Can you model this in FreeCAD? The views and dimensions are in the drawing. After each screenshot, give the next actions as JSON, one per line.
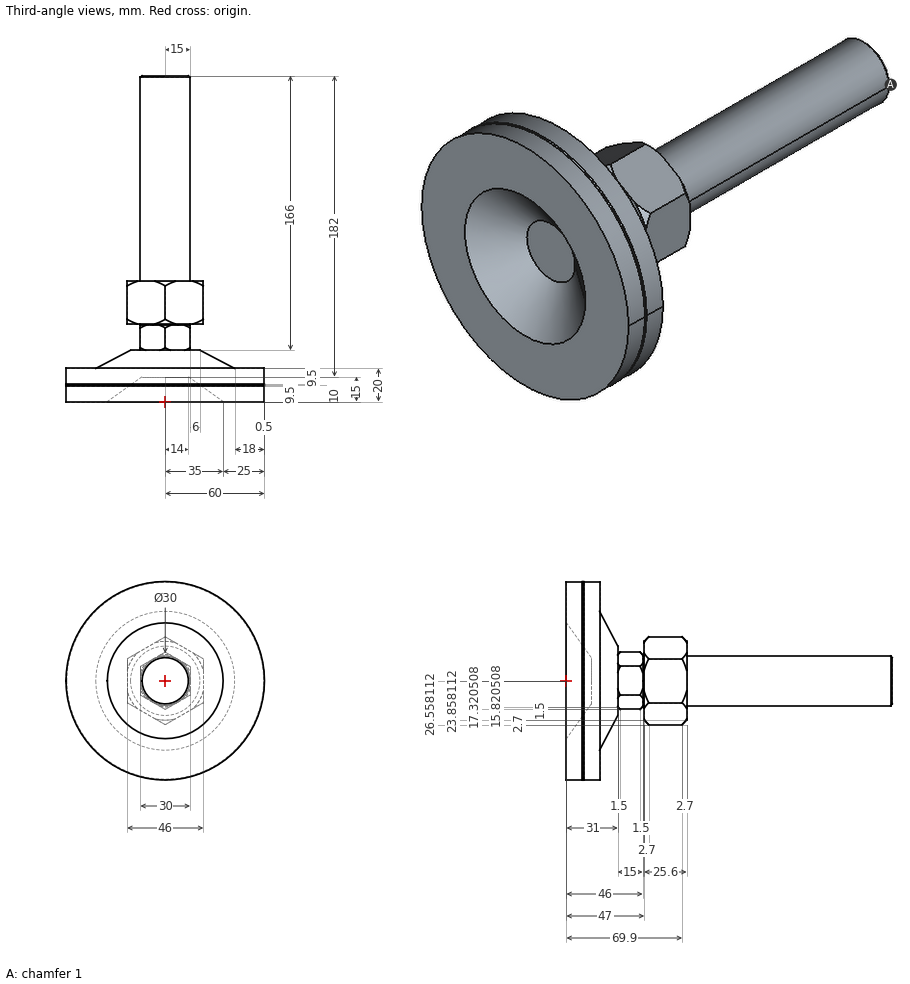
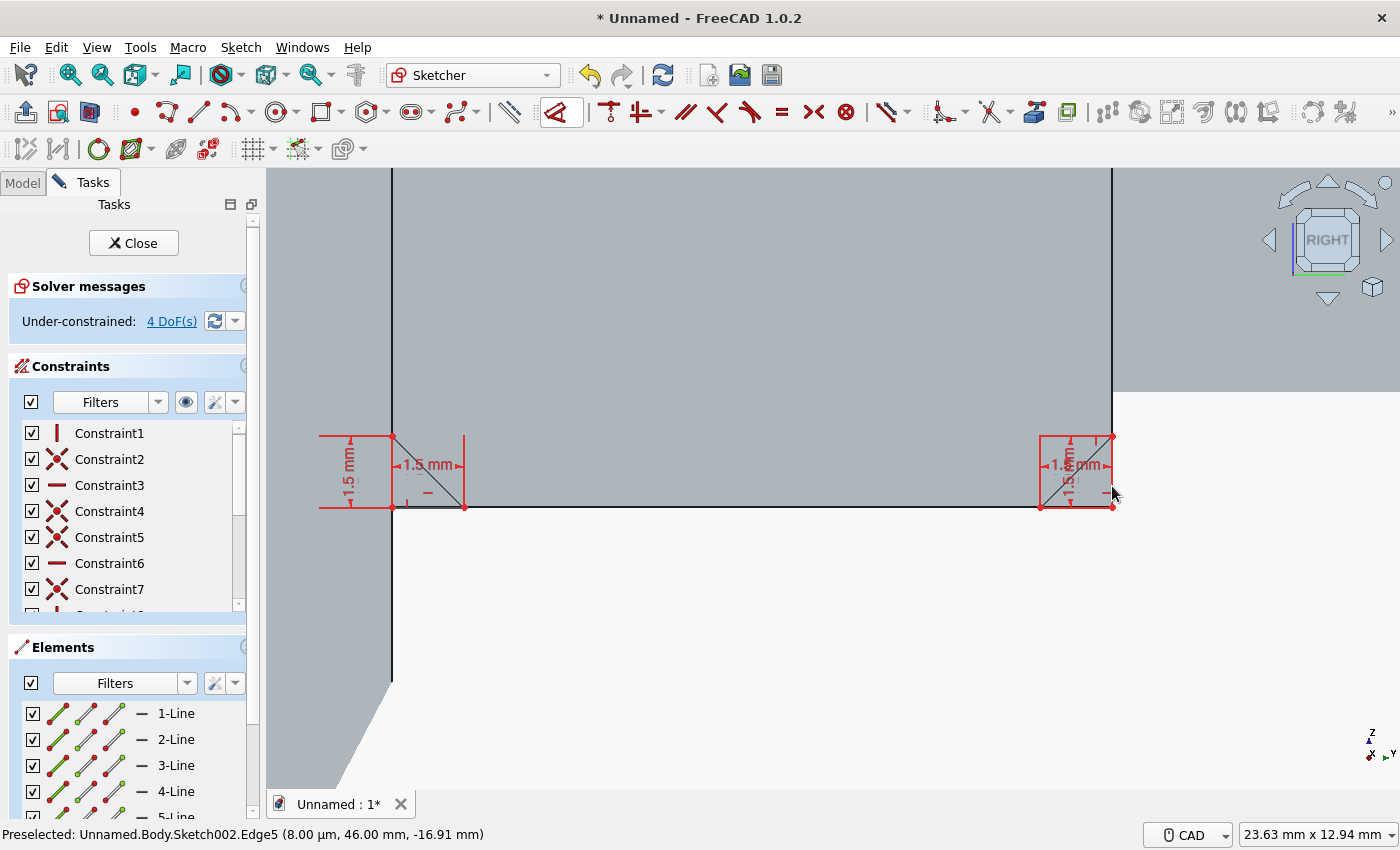
{"action": "left_click", "coordinate": [392, 436]}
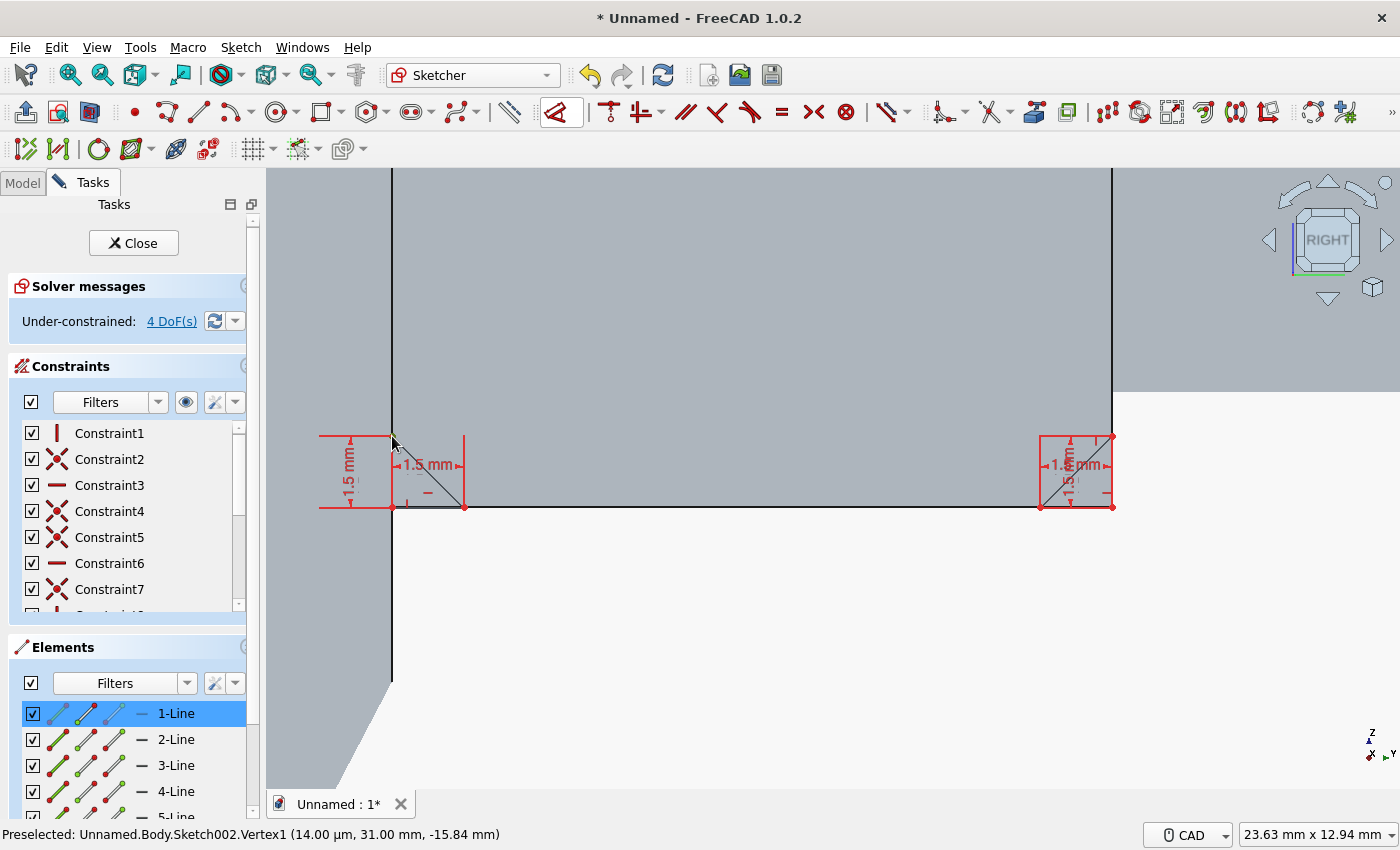
{"action": "key", "text": "l"}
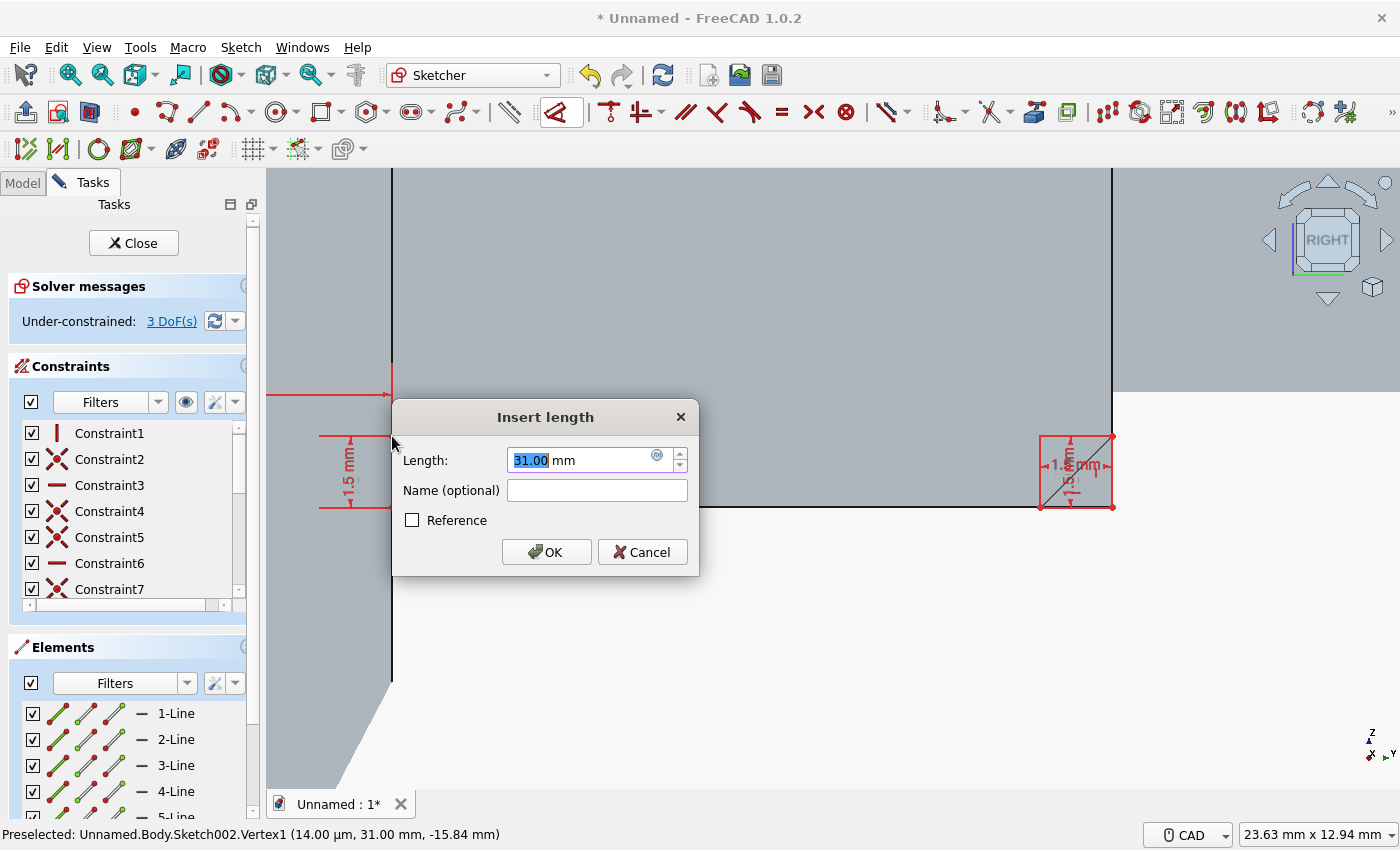
{"action": "type", "text": "31"}
{"action": "key", "text": "Return"}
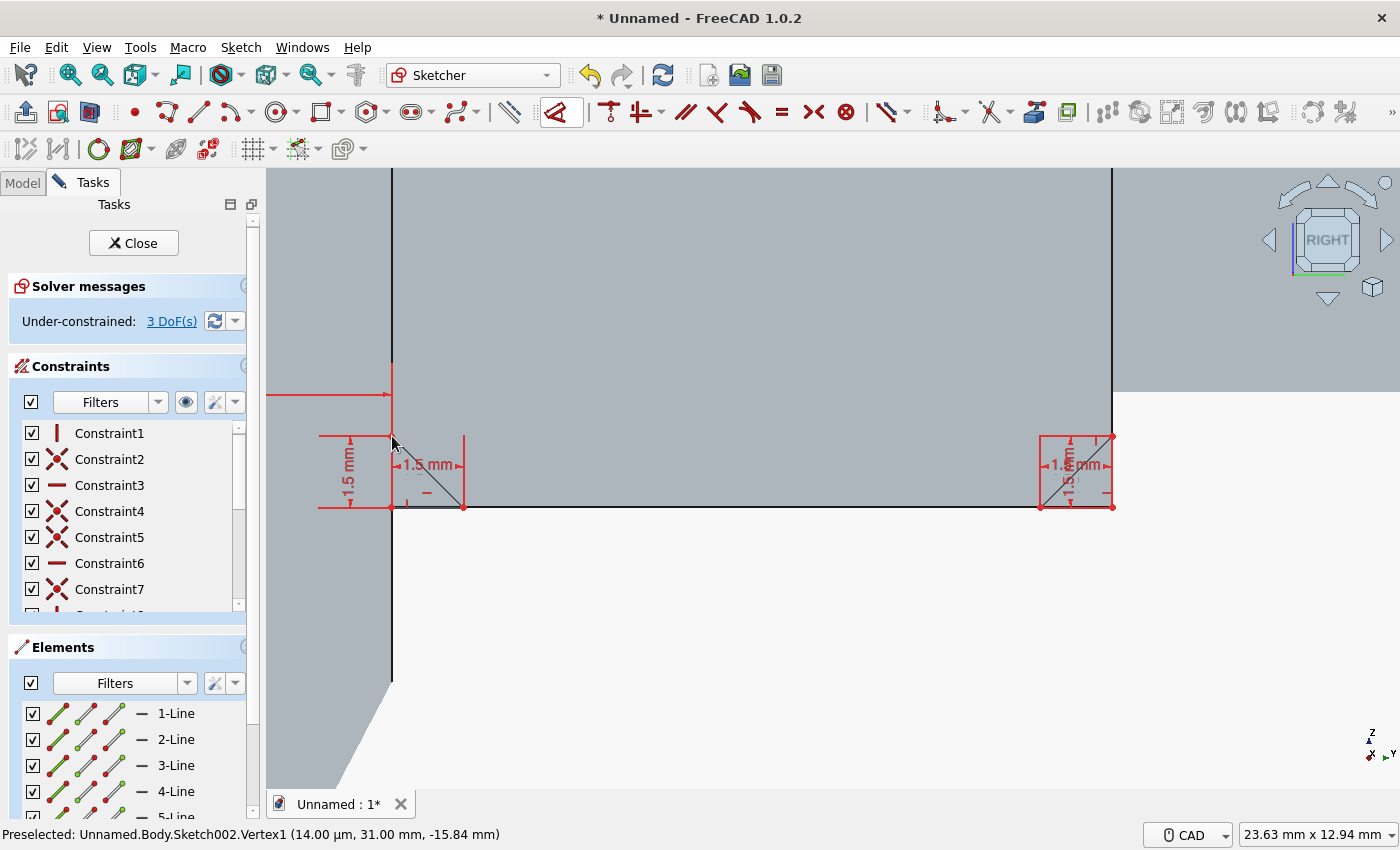
{"action": "left_click", "coordinate": [1112, 508]}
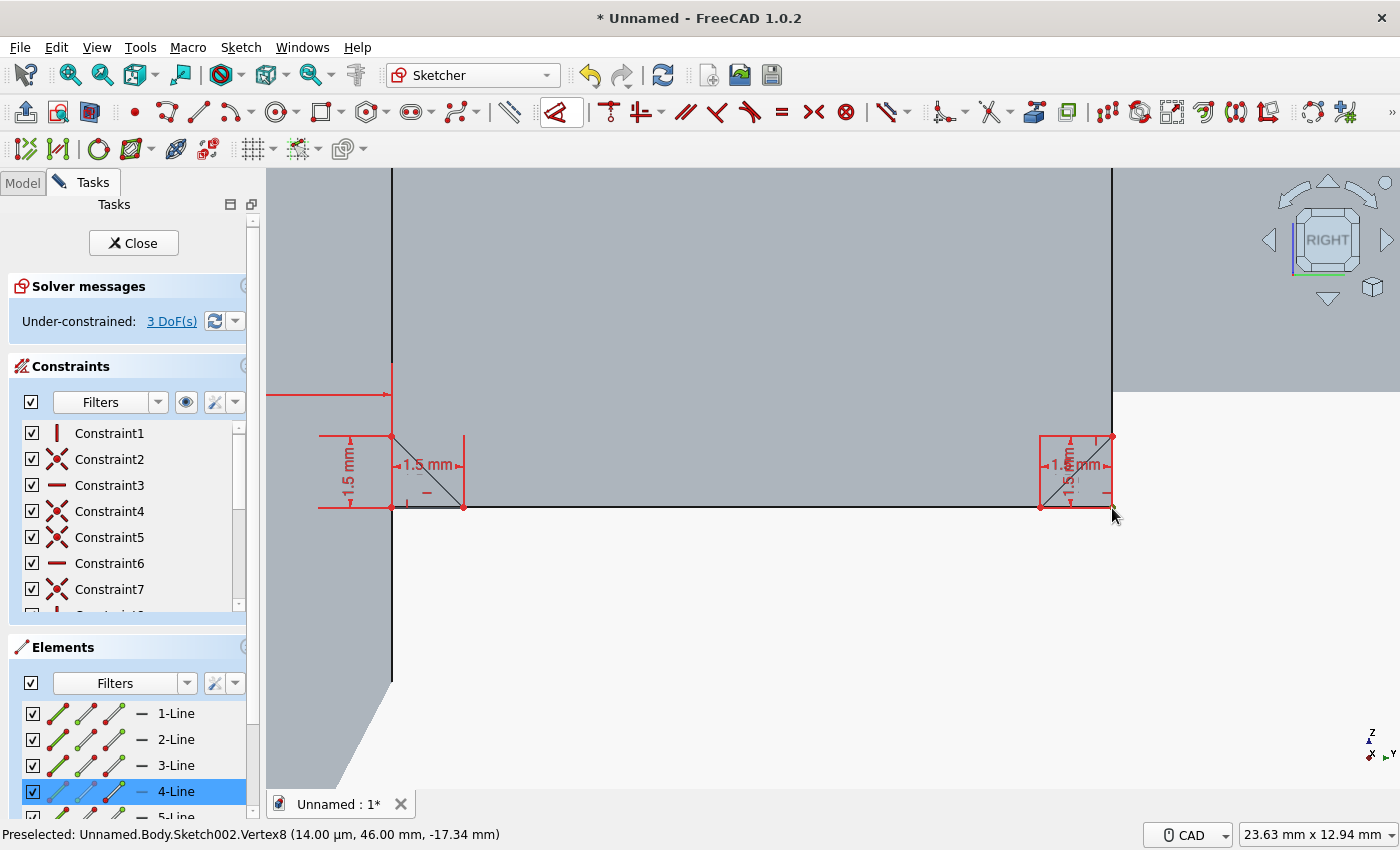
{"action": "key", "text": "l"}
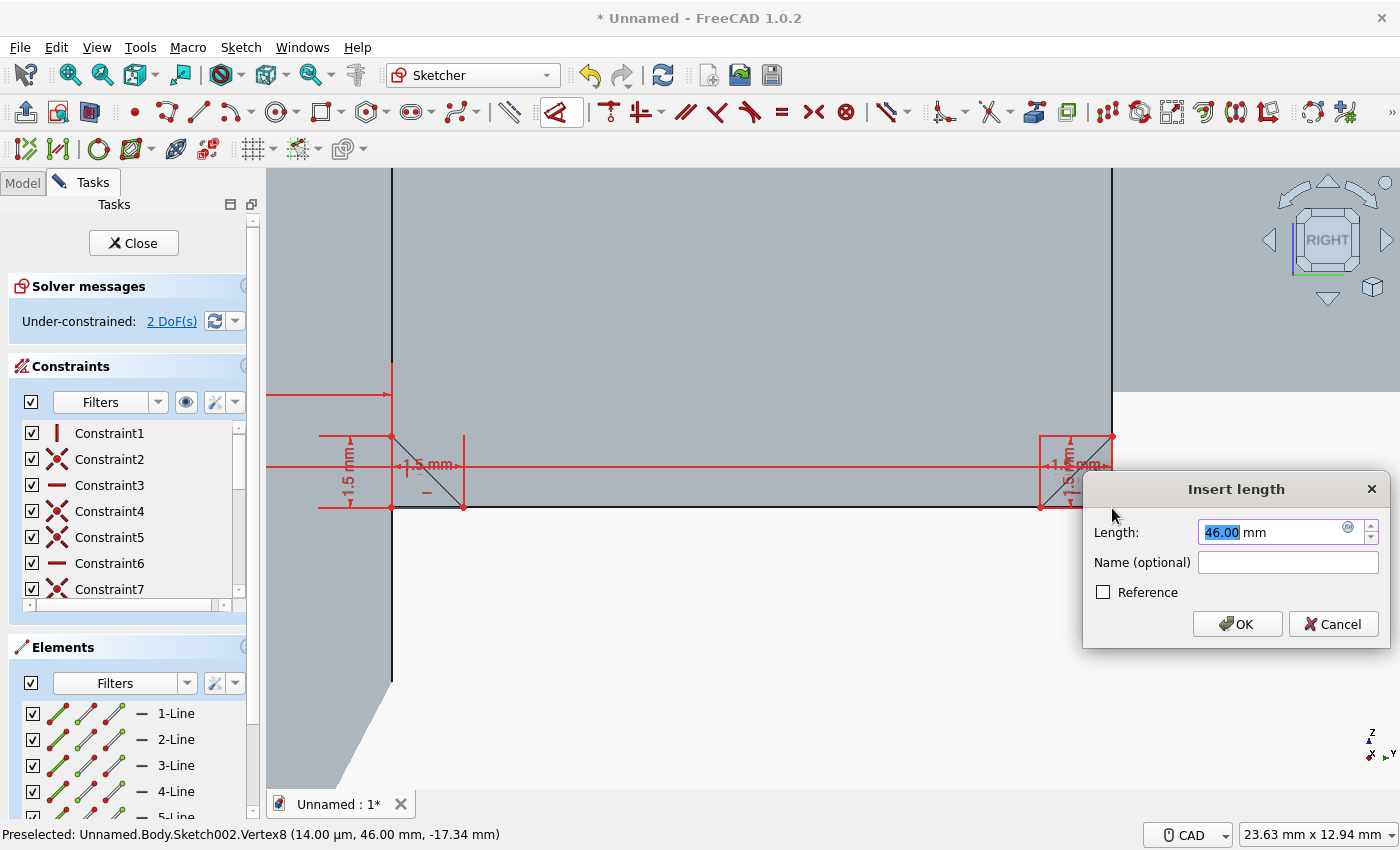
{"action": "type", "text": "46"}
{"action": "key", "text": "Return"}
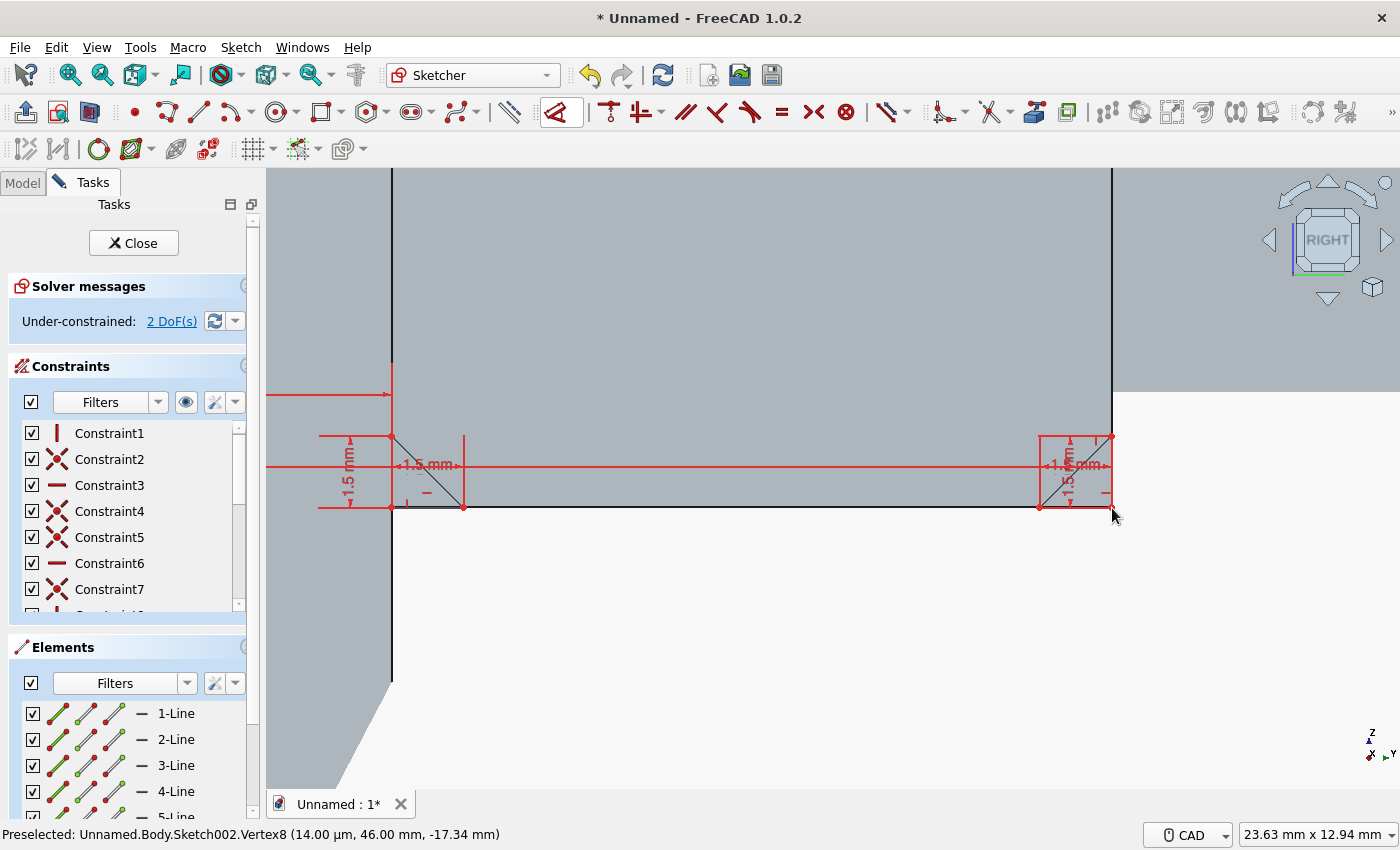
{"action": "left_click", "coordinate": [392, 436]}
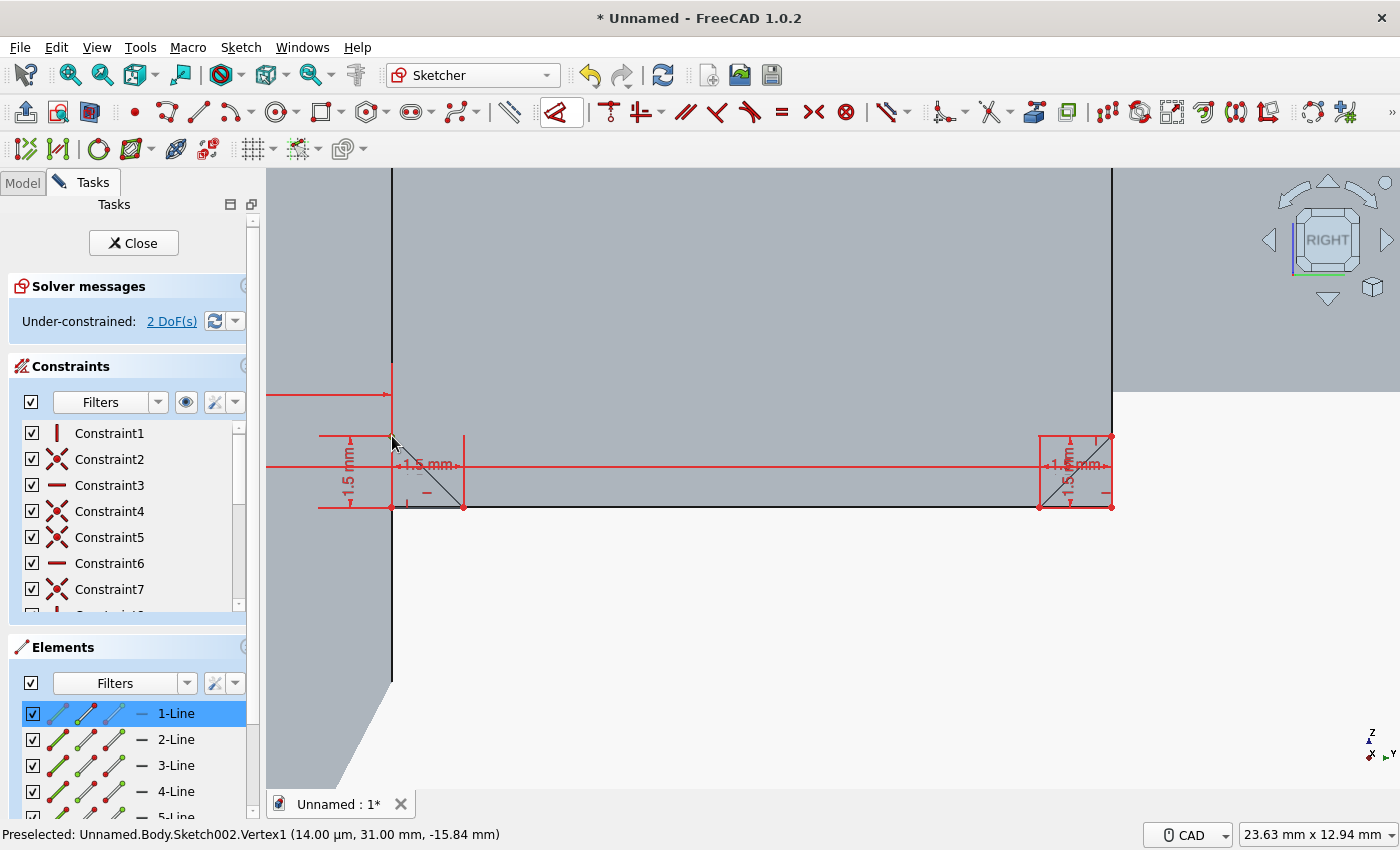
{"action": "key", "text": "i"}